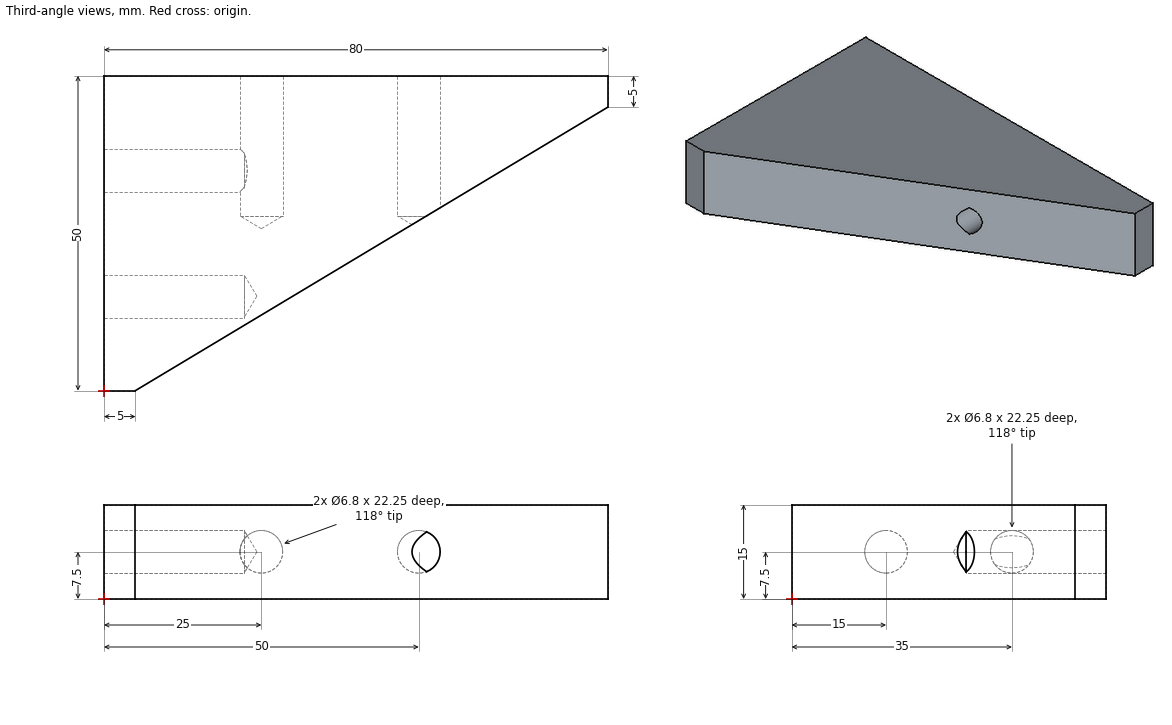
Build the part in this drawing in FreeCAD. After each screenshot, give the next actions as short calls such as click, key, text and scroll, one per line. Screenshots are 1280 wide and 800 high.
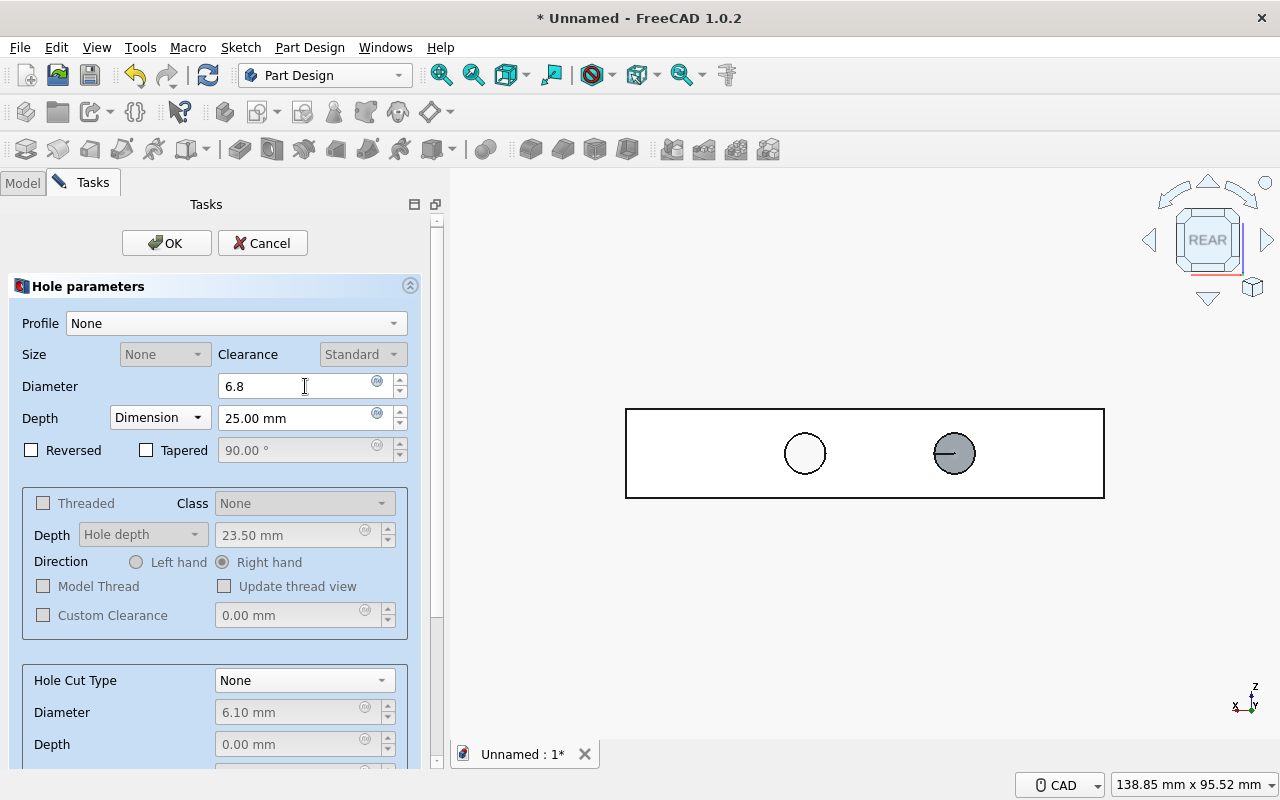
triple_click(305, 418)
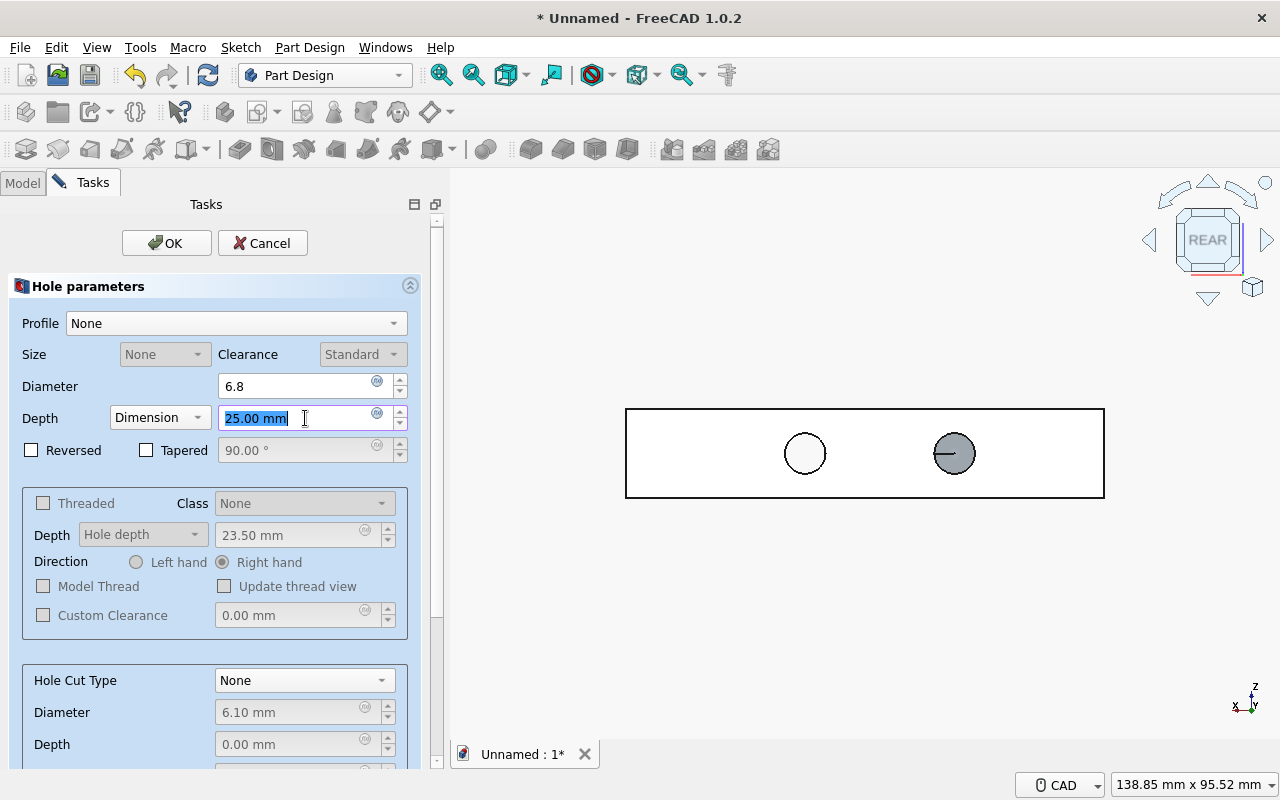
text(22.25)
key(Tab)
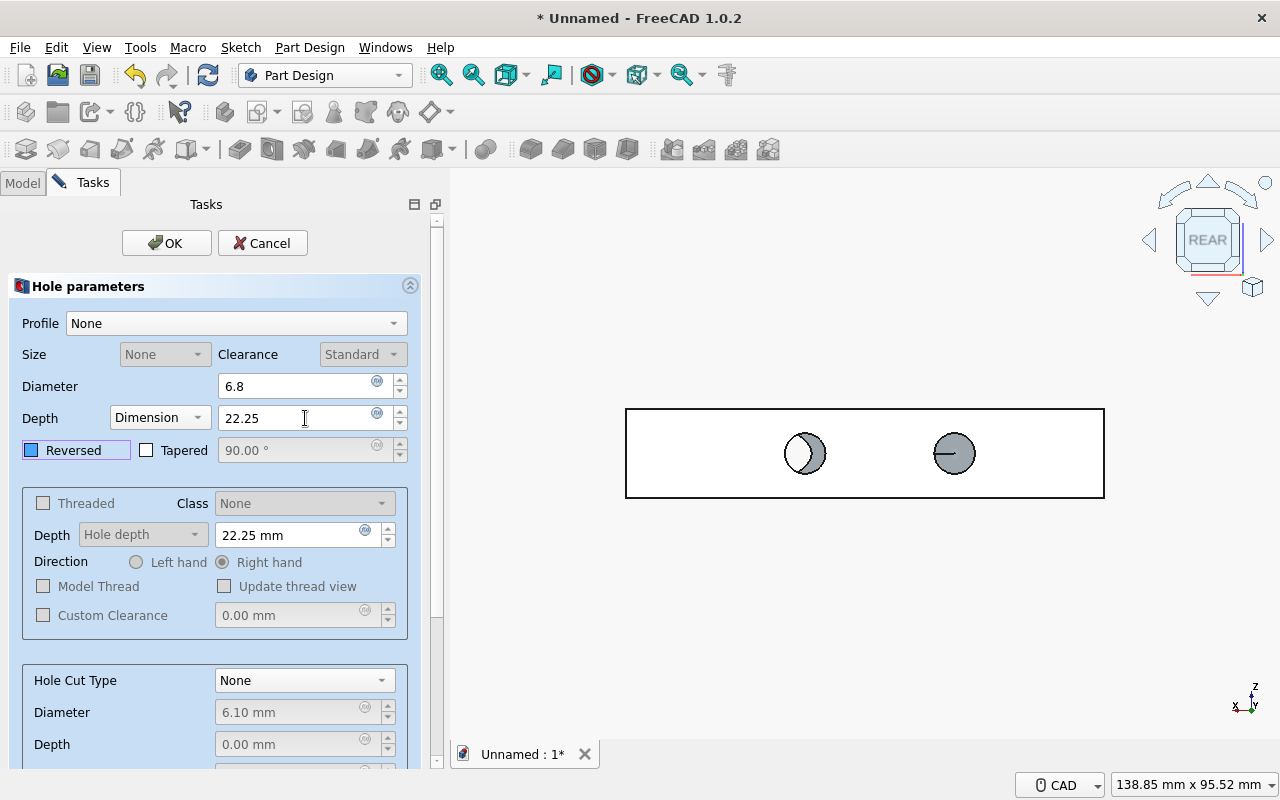
click(167, 243)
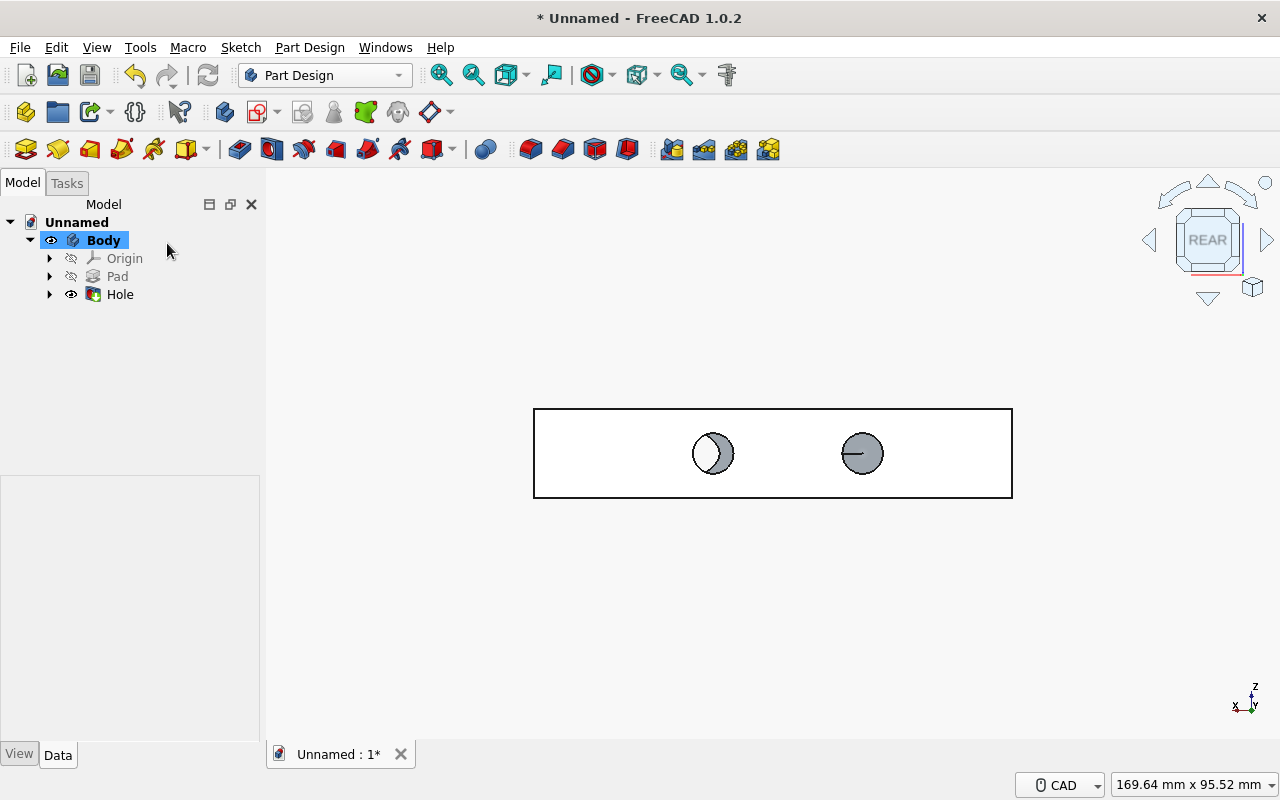
key(6)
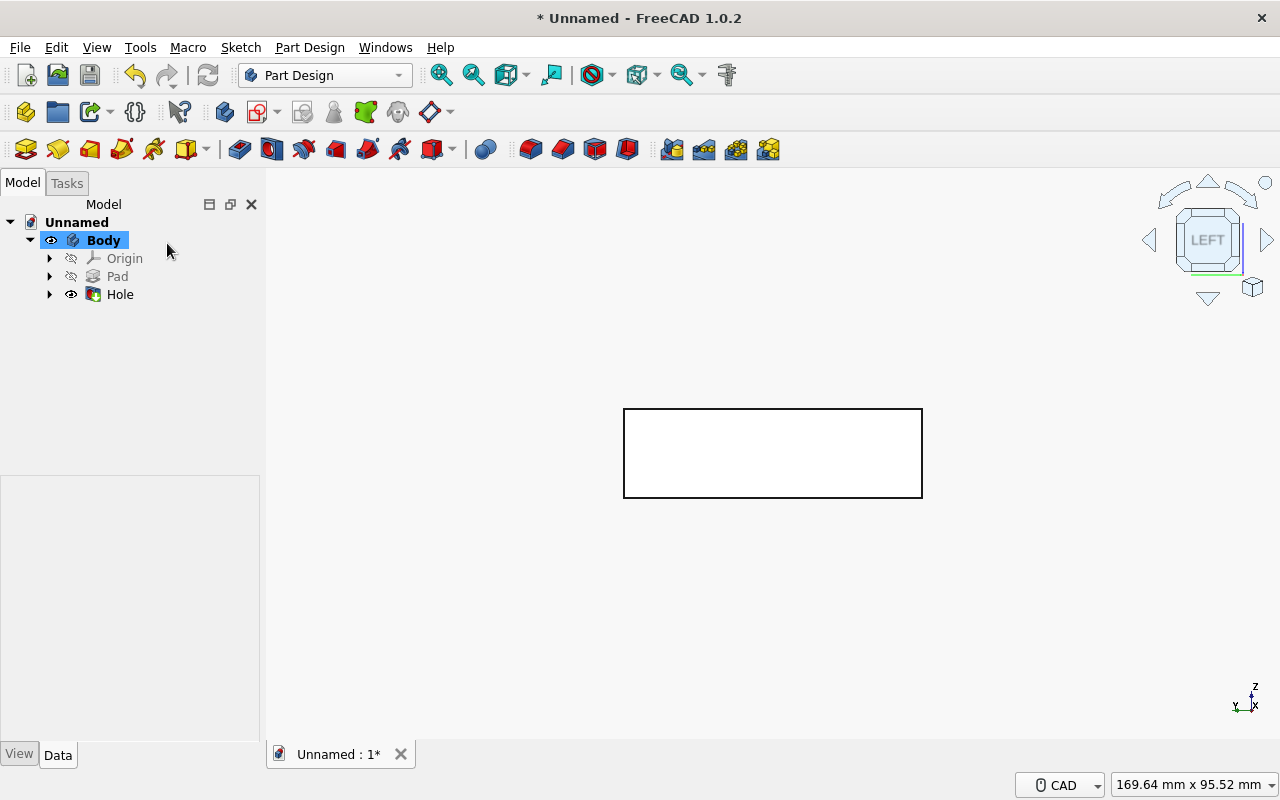
key(v)
key(f)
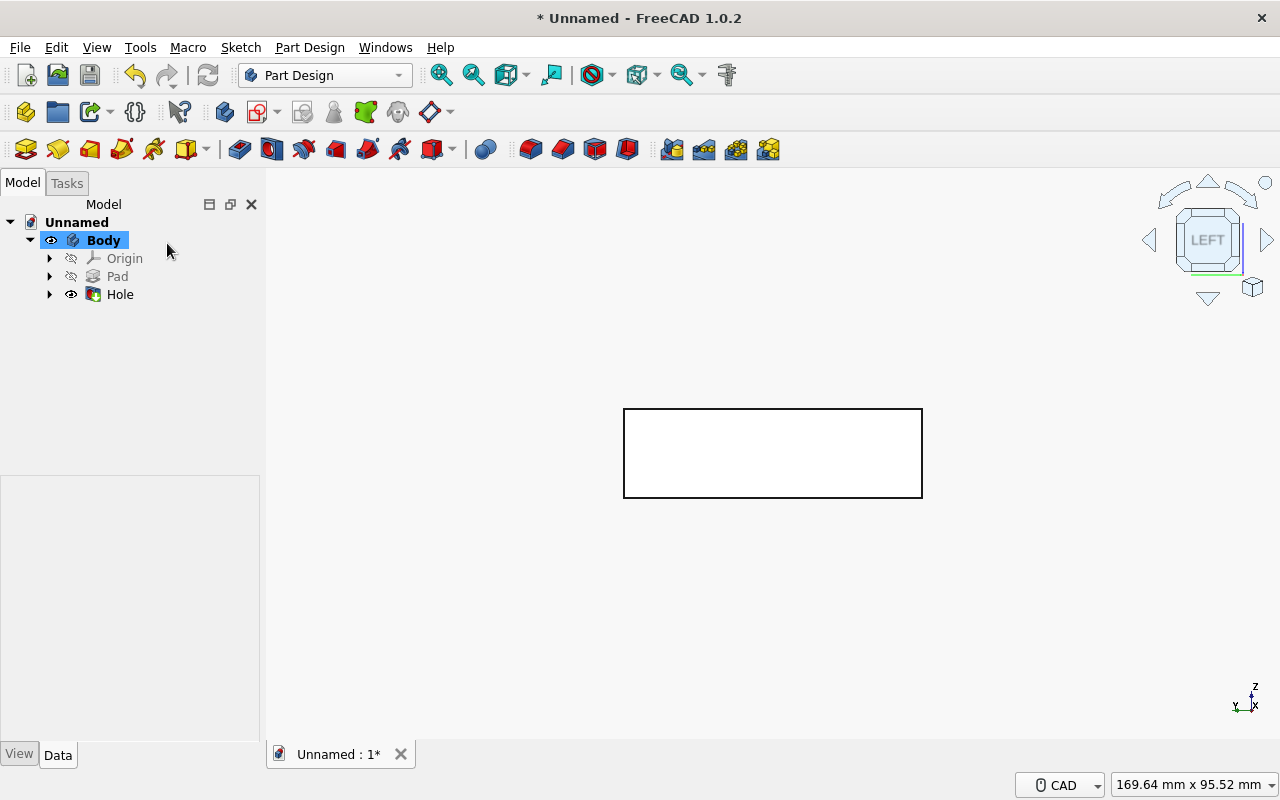
click(688, 452)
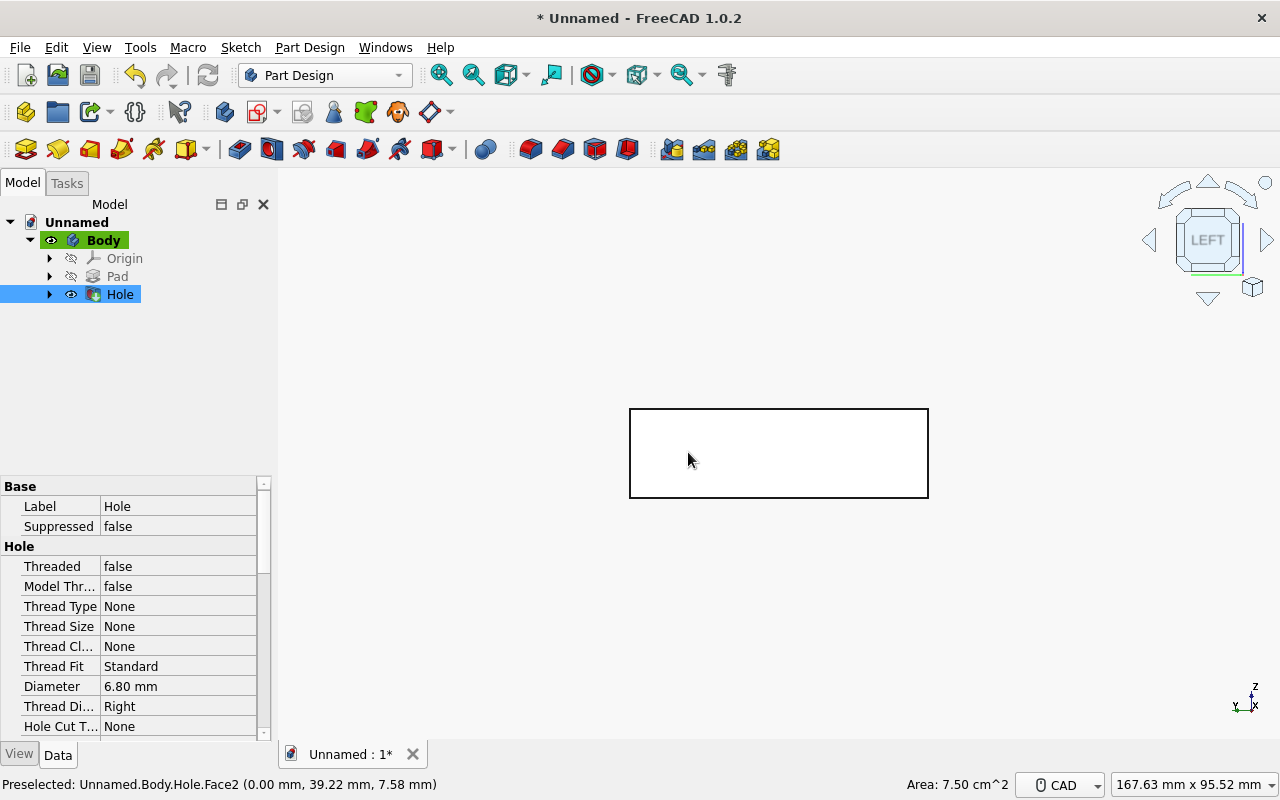
click(258, 112)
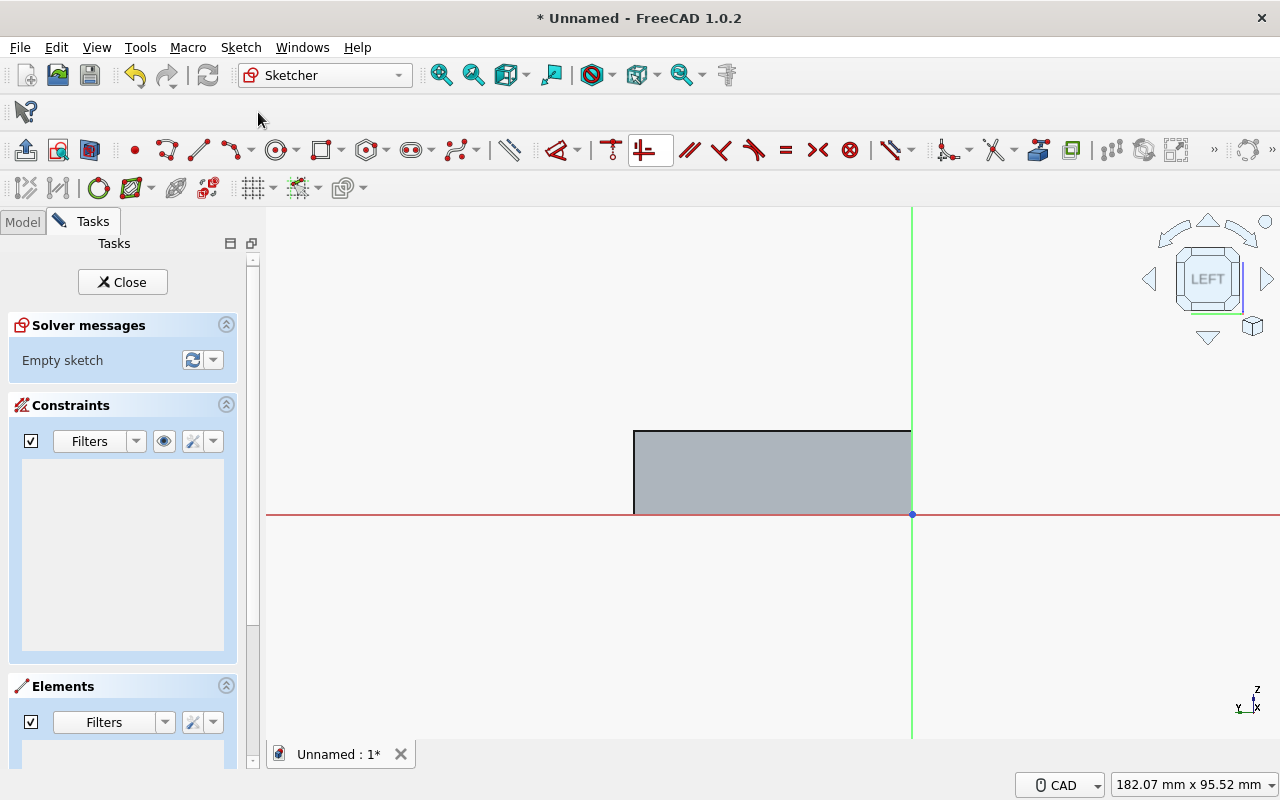
scroll(864, 491, up, 5)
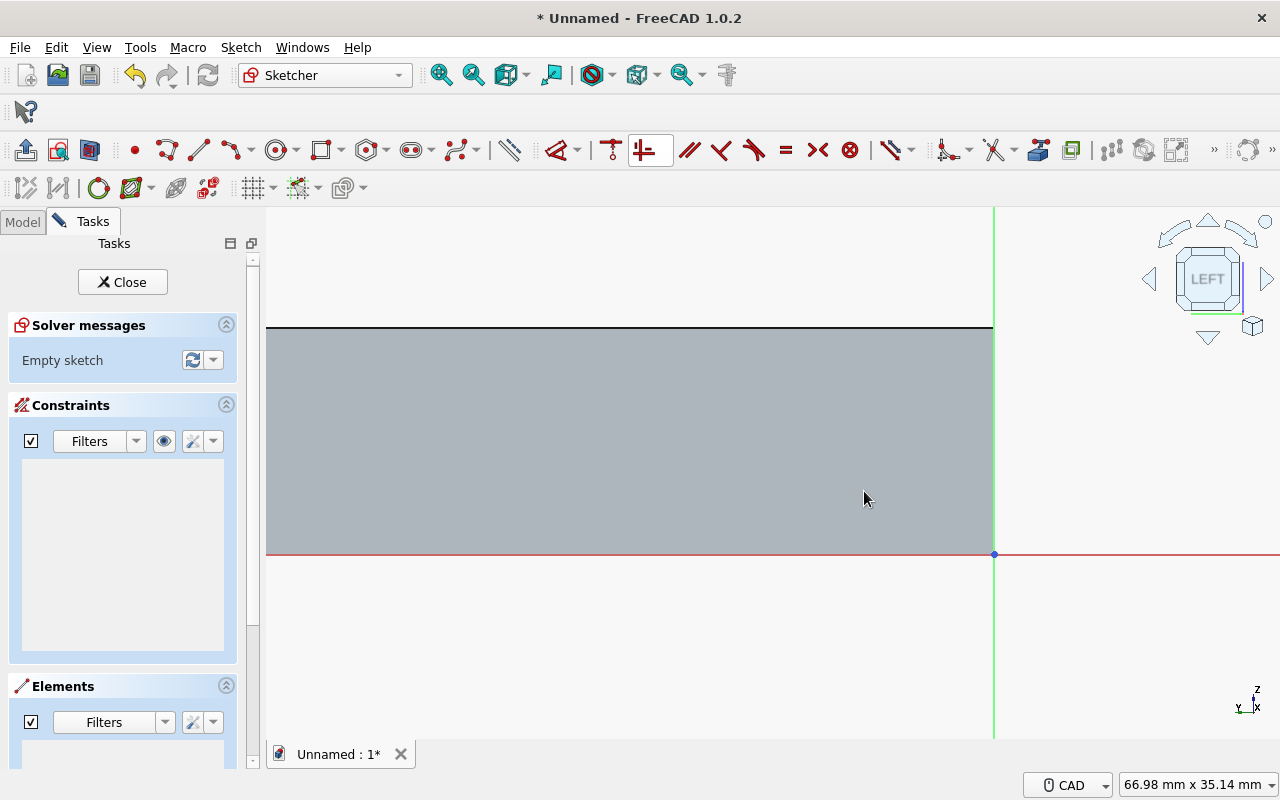
key(g)
key(c)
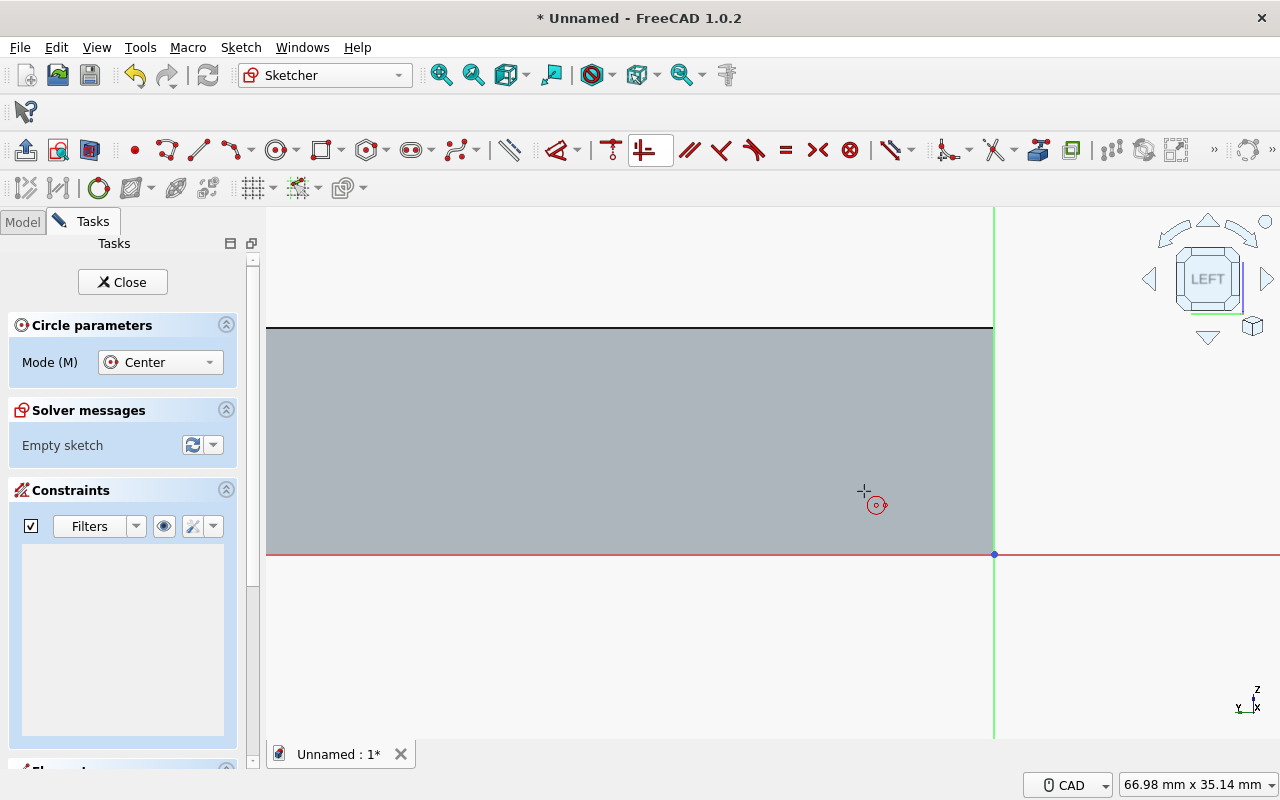
click(464, 441)
move(501, 405)